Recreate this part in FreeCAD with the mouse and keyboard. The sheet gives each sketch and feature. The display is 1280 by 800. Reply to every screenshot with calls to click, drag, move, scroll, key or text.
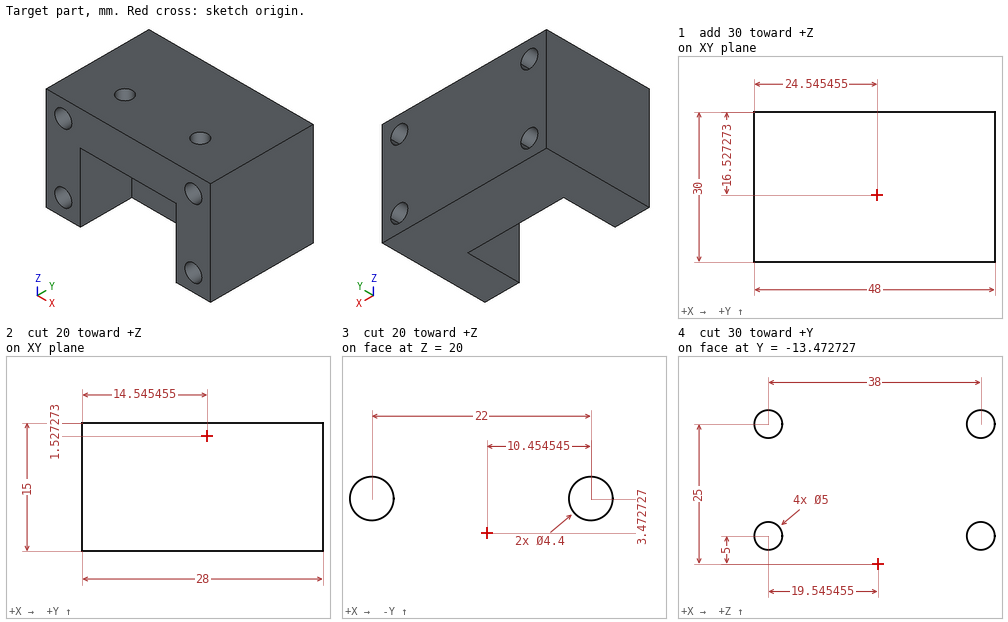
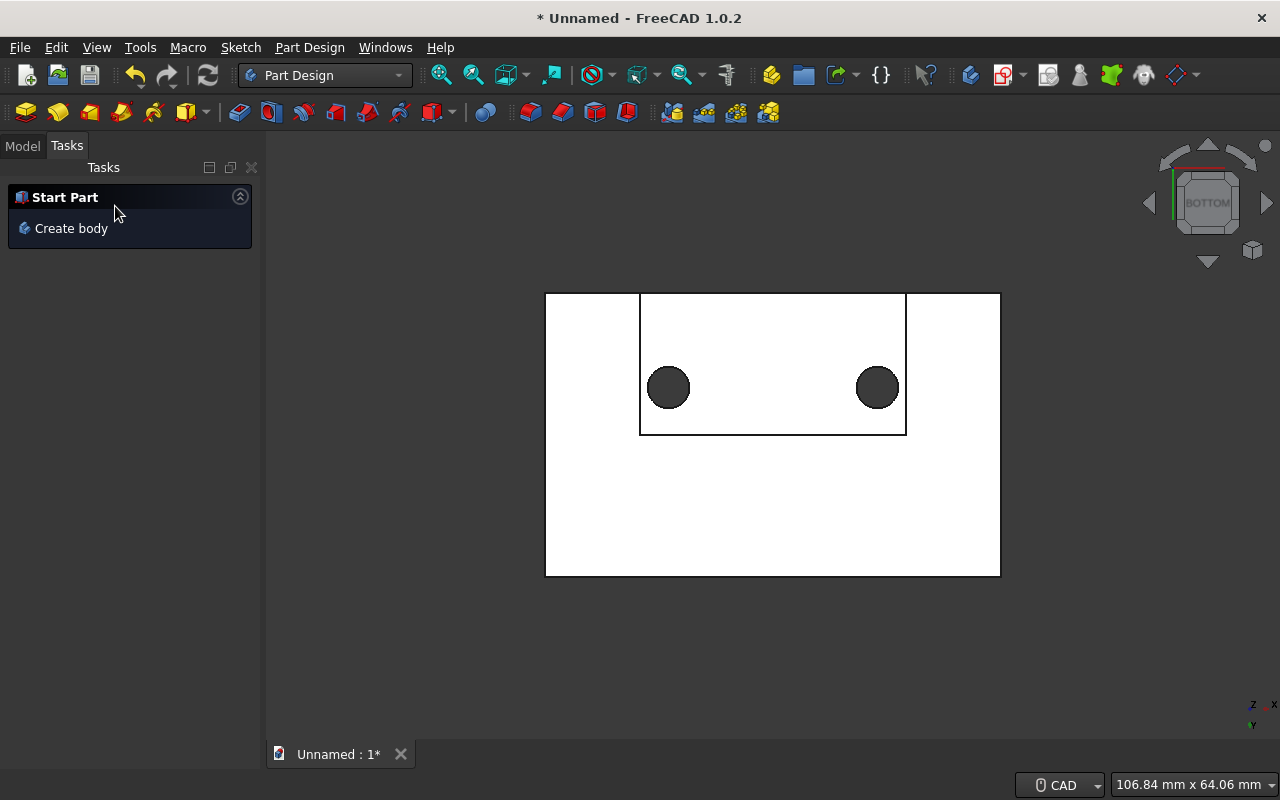
key(0)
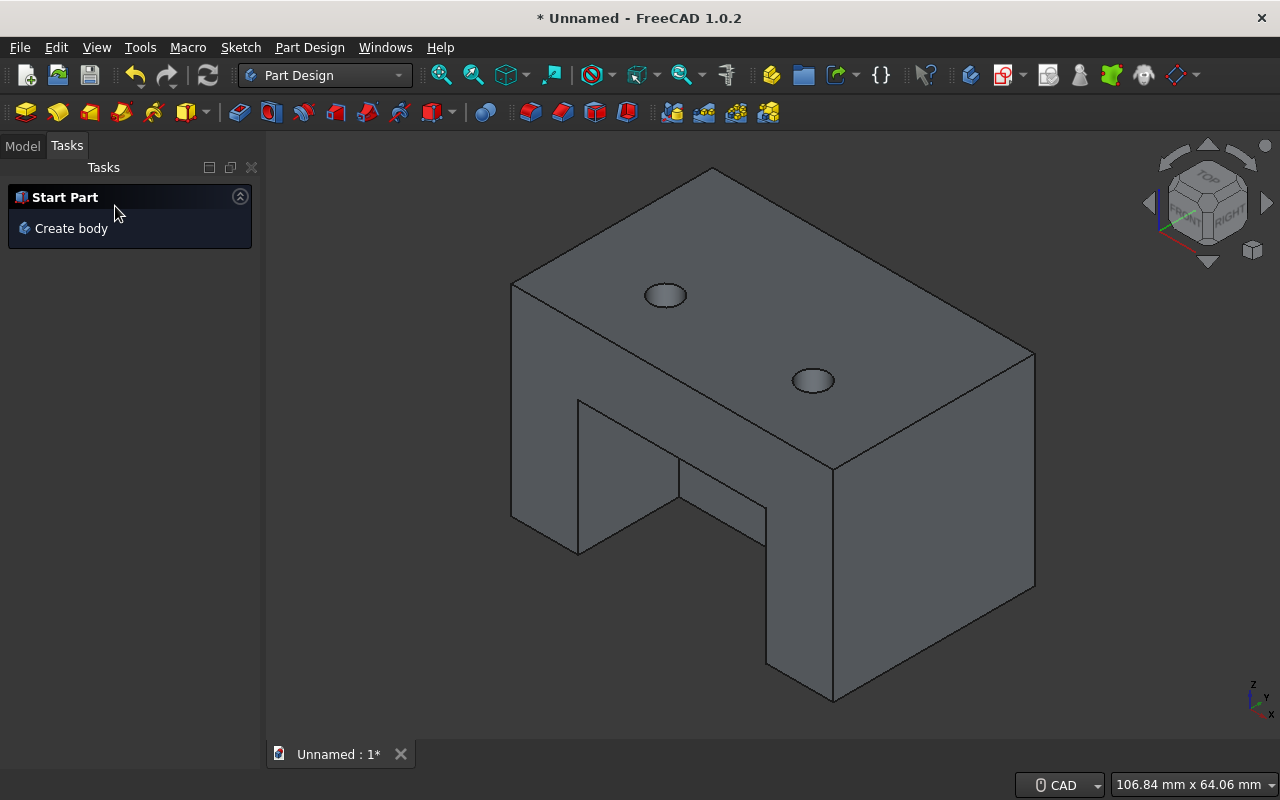
click(764, 479)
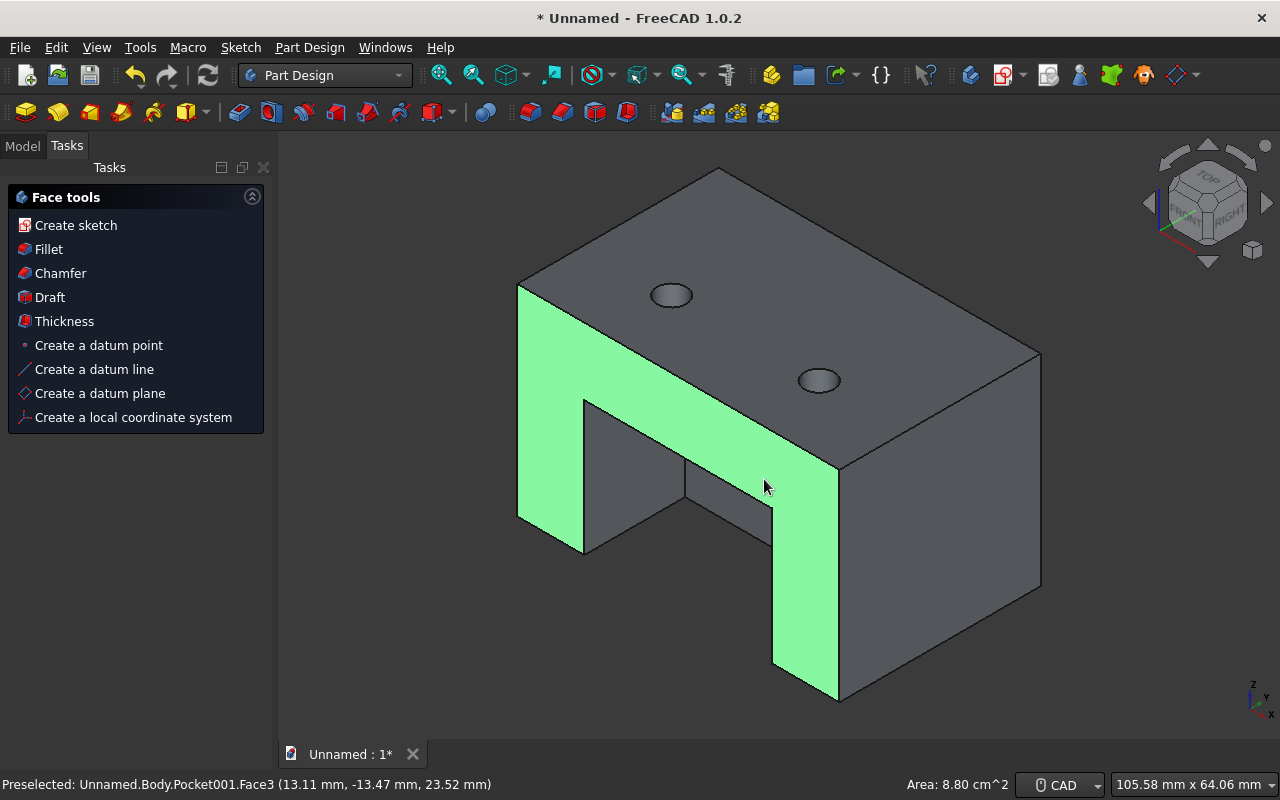
click(1004, 76)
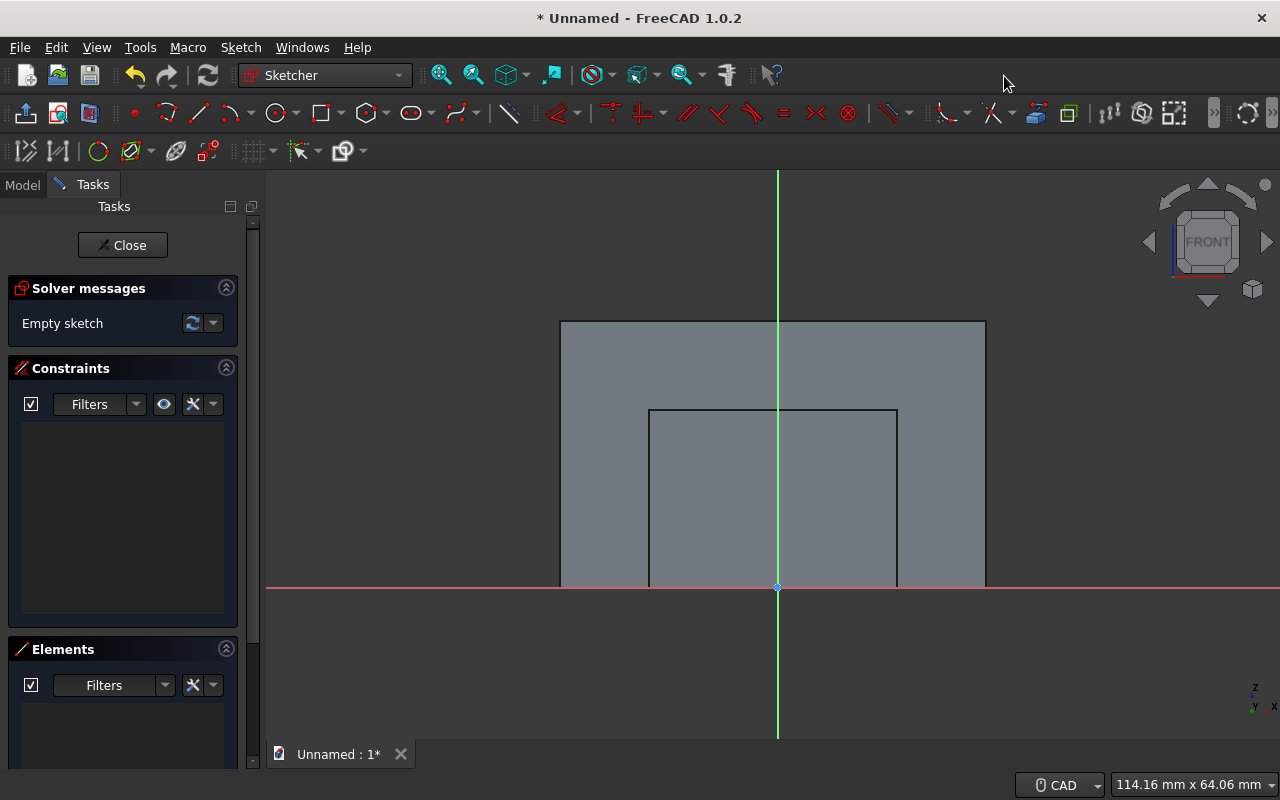
scroll(912, 488, up, 2)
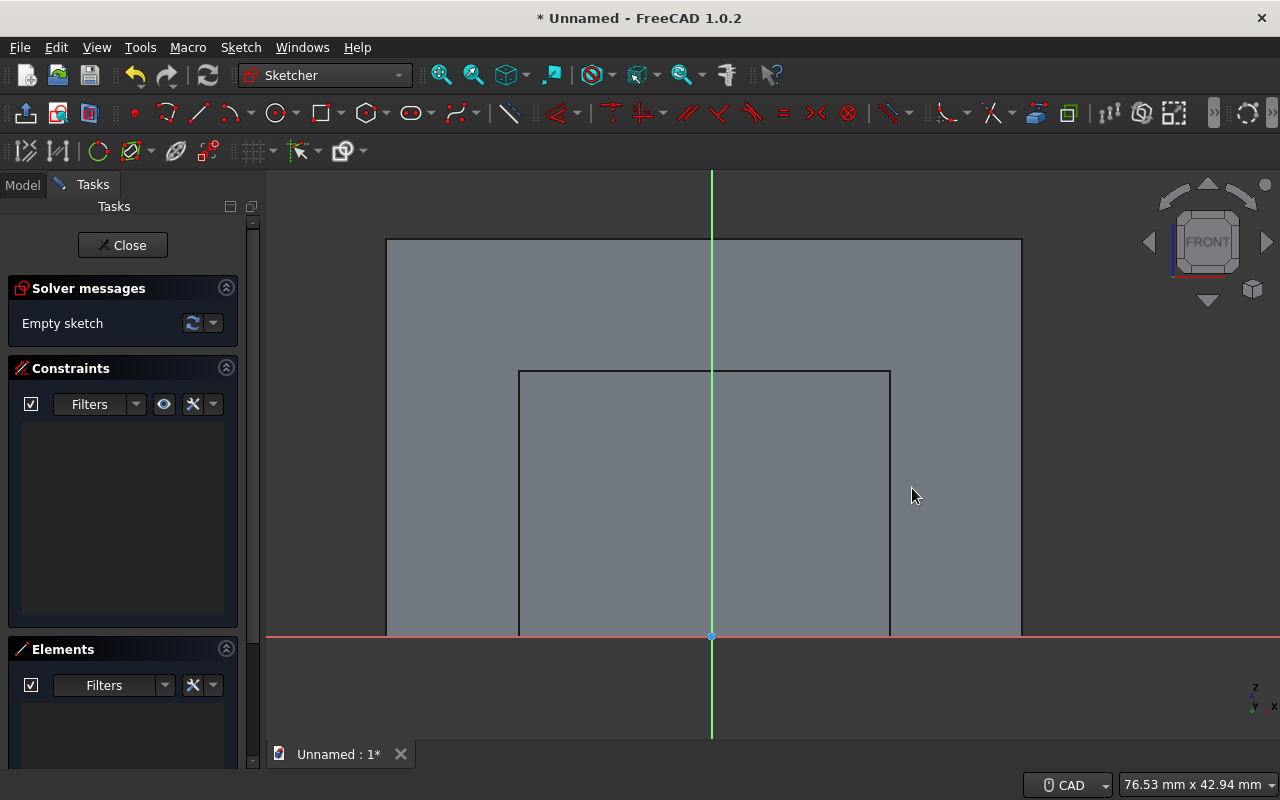
click(276, 114)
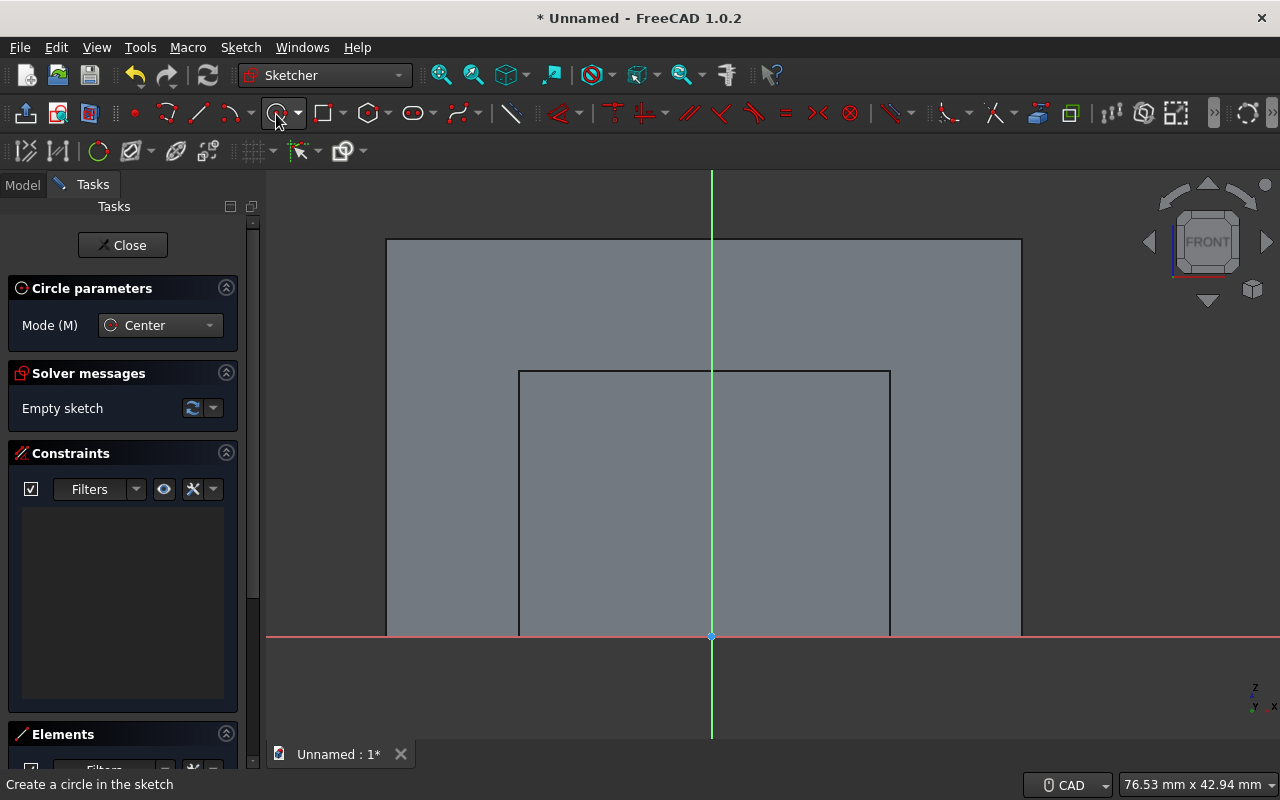
click(453, 570)
click(476, 547)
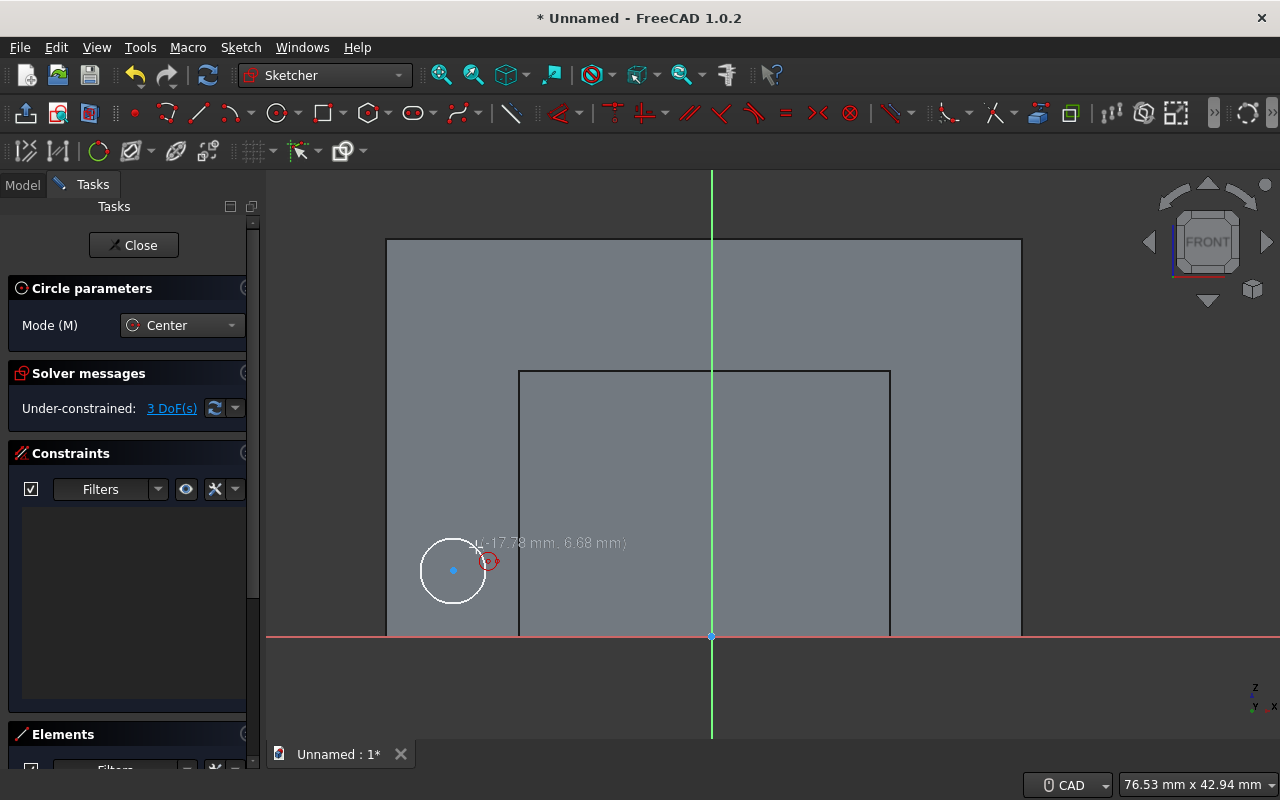
click(453, 305)
click(476, 282)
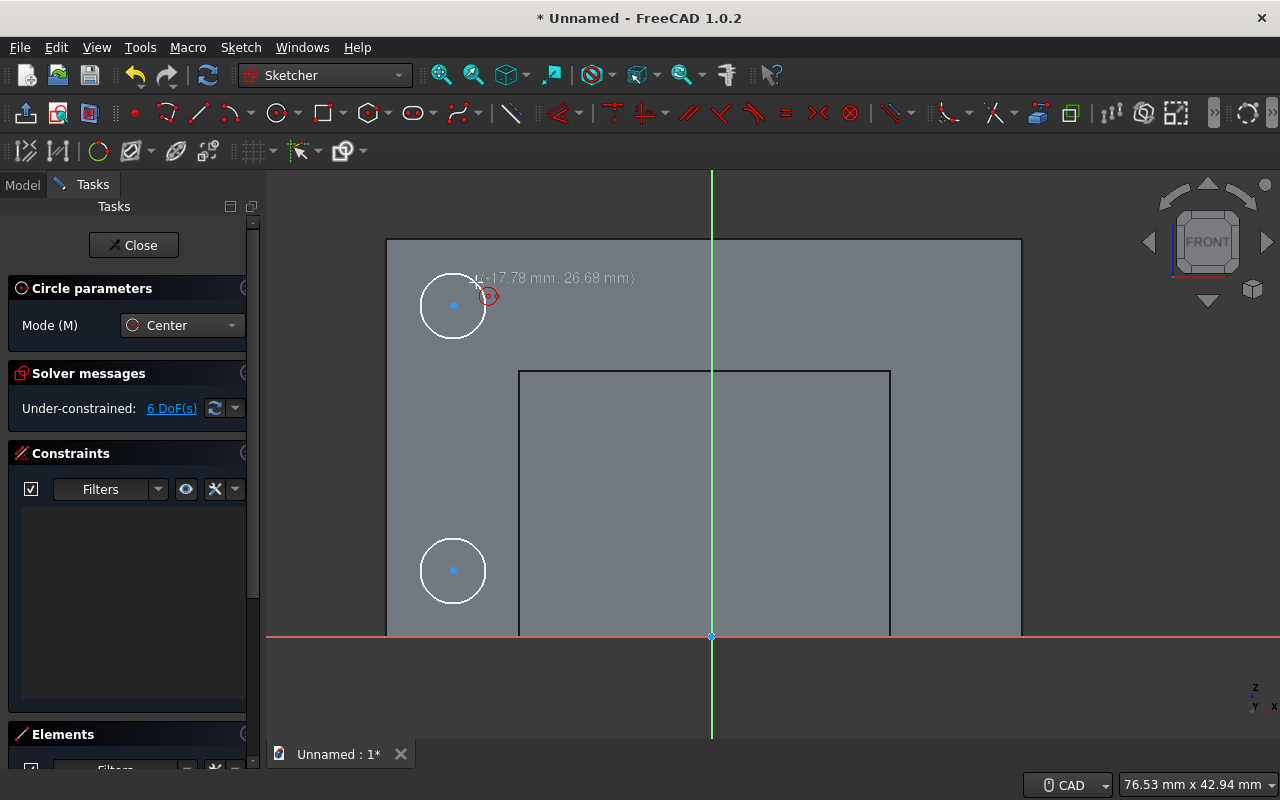
click(956, 305)
click(980, 282)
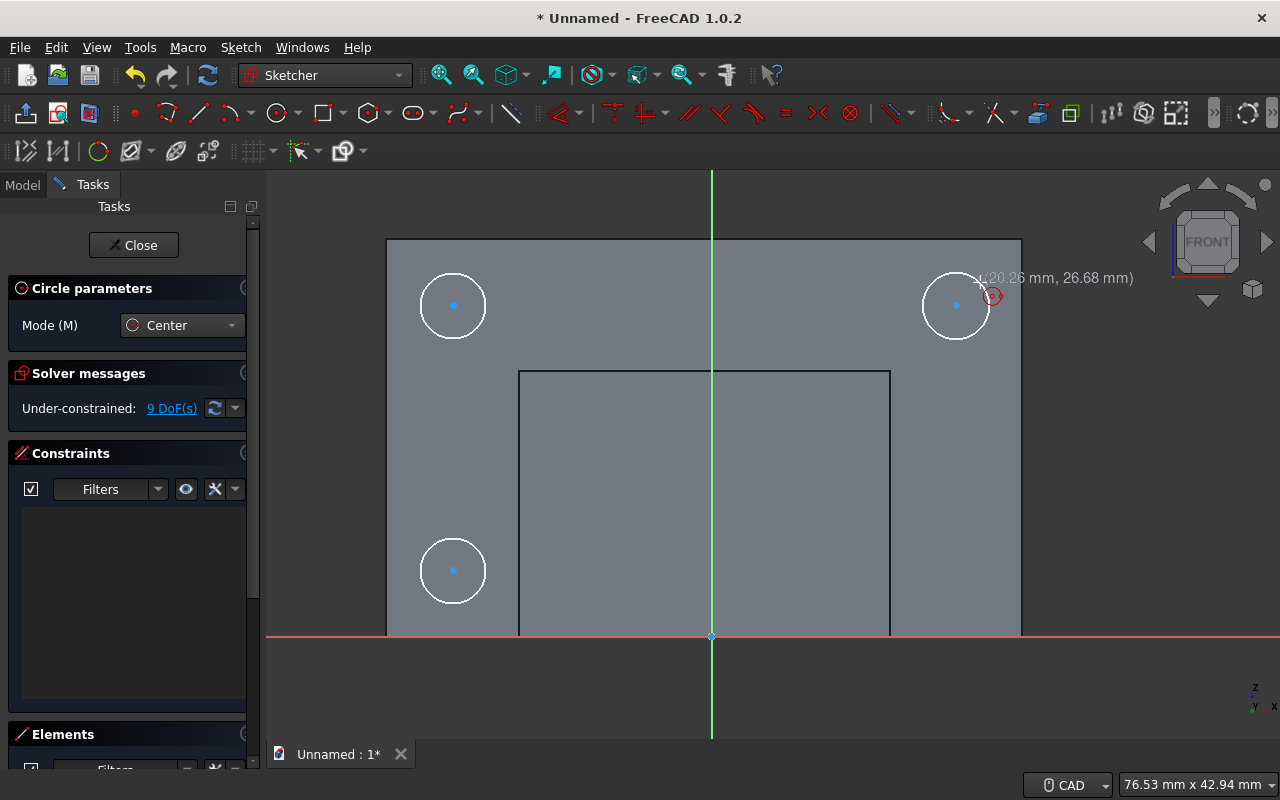
click(956, 570)
click(980, 547)
key(Escape)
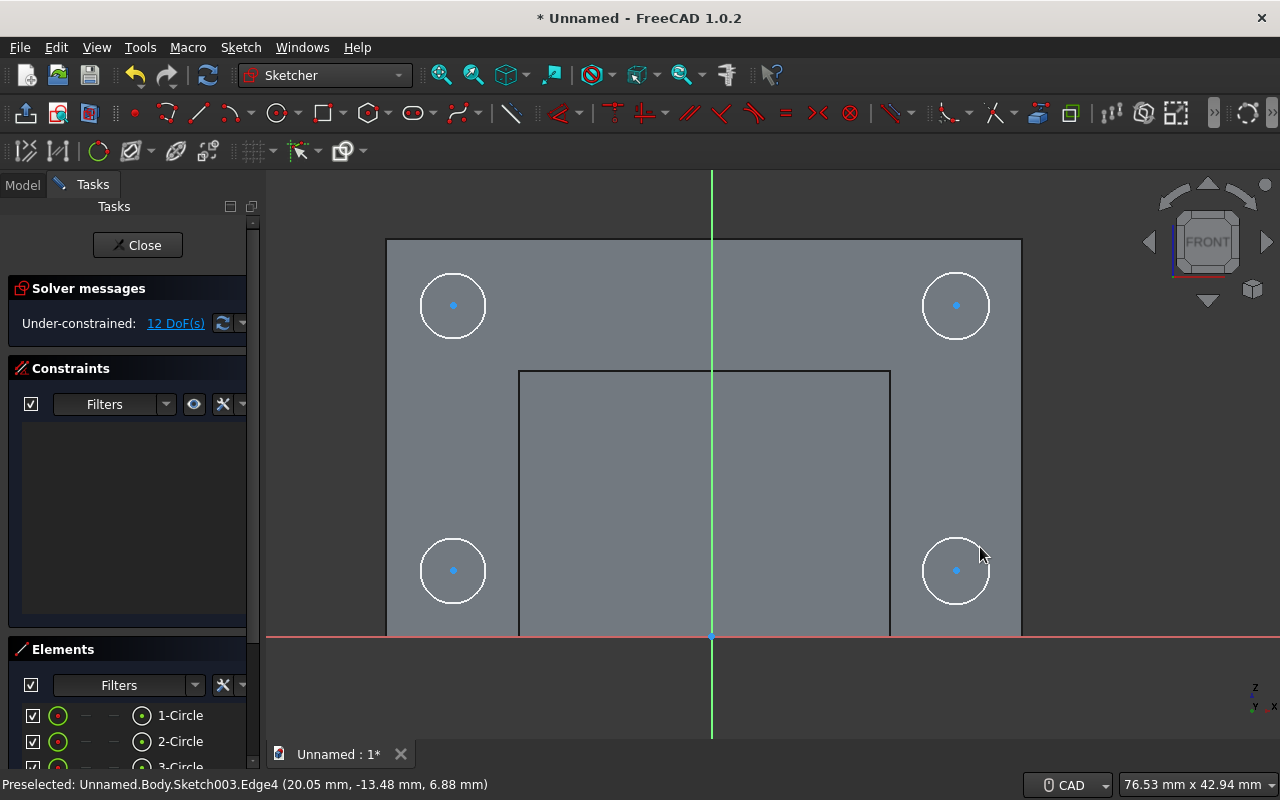
click(476, 548)